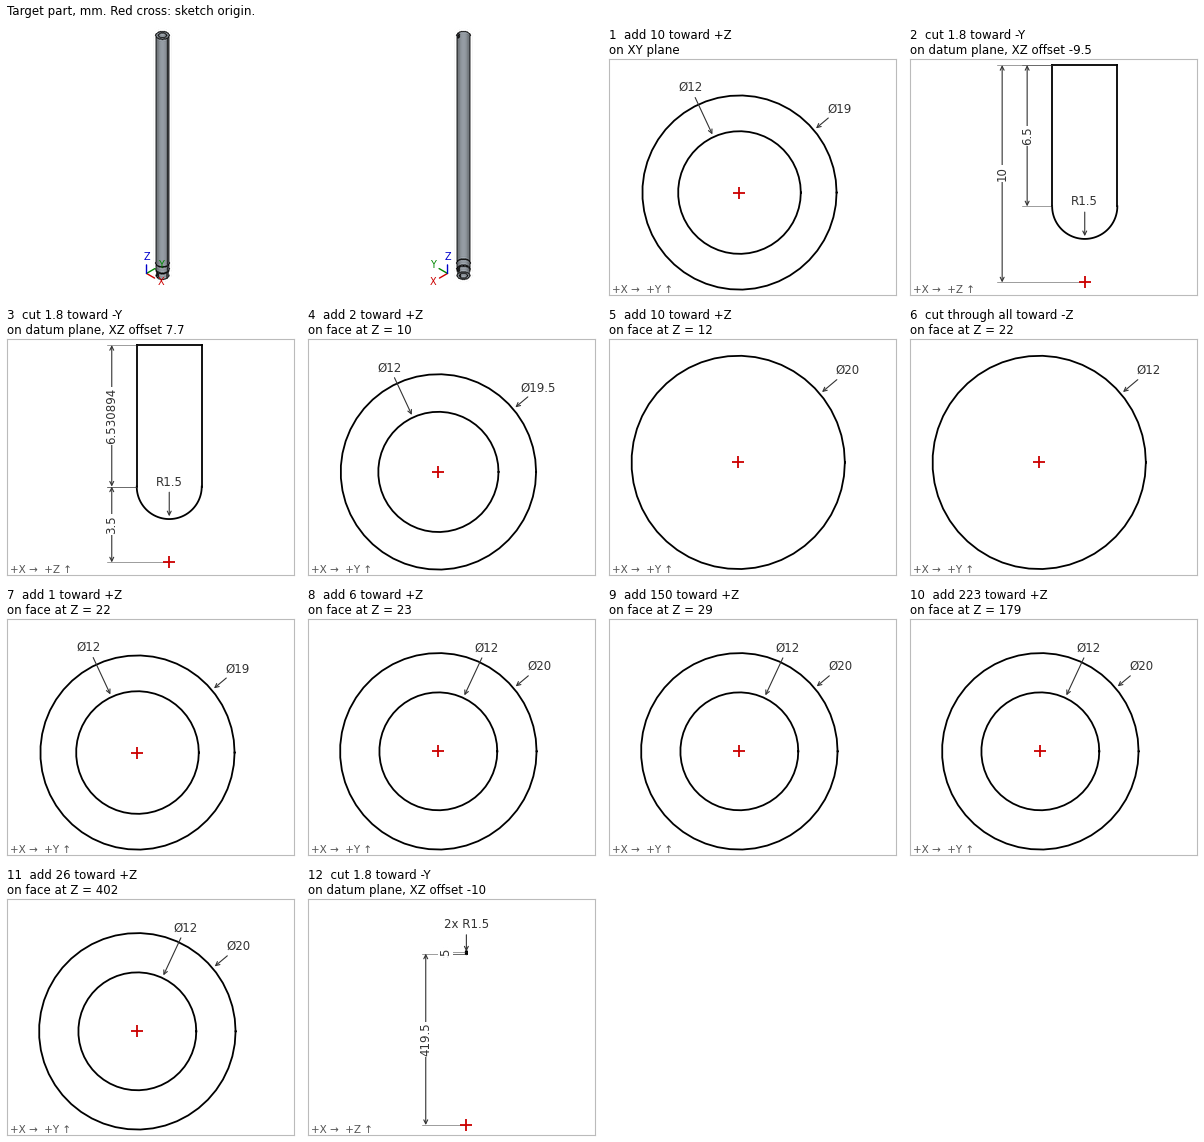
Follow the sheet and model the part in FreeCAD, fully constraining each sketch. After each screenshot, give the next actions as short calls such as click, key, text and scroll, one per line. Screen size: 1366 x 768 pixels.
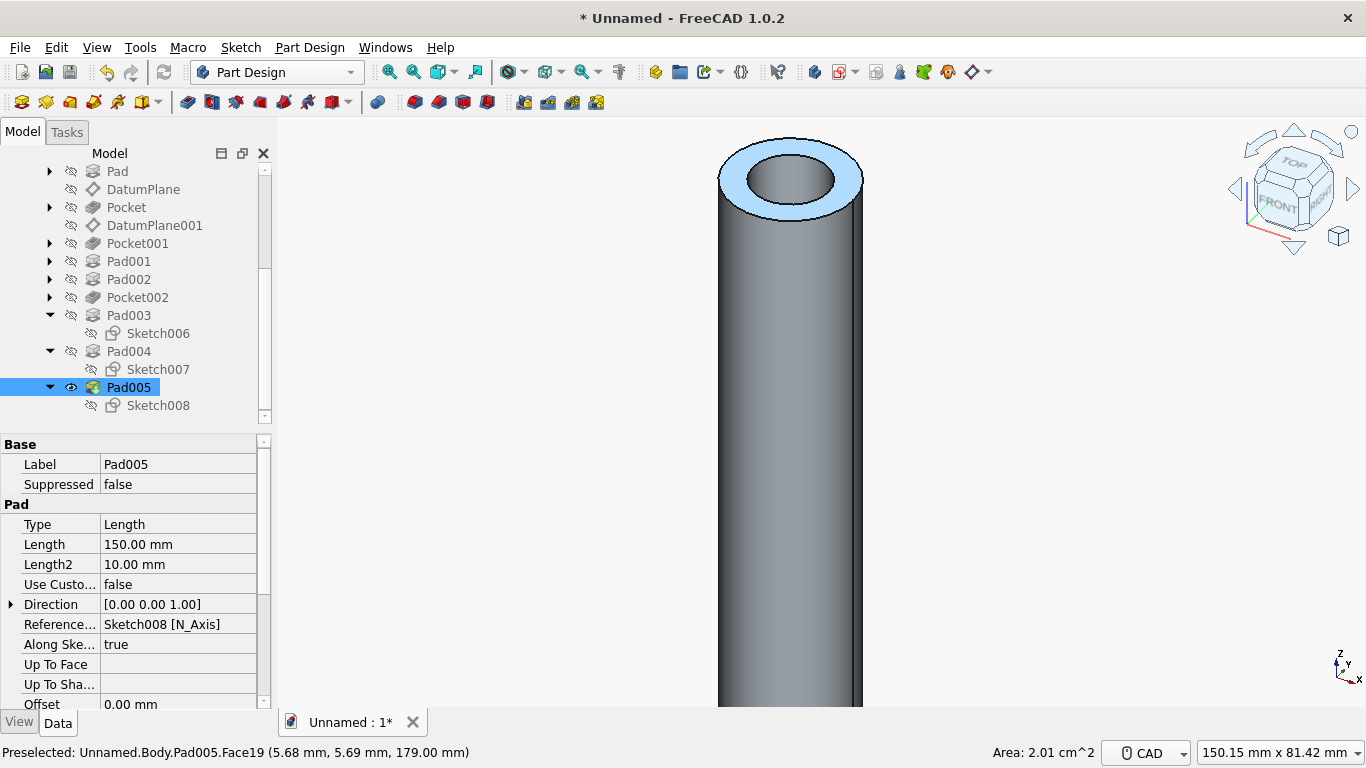
click(840, 72)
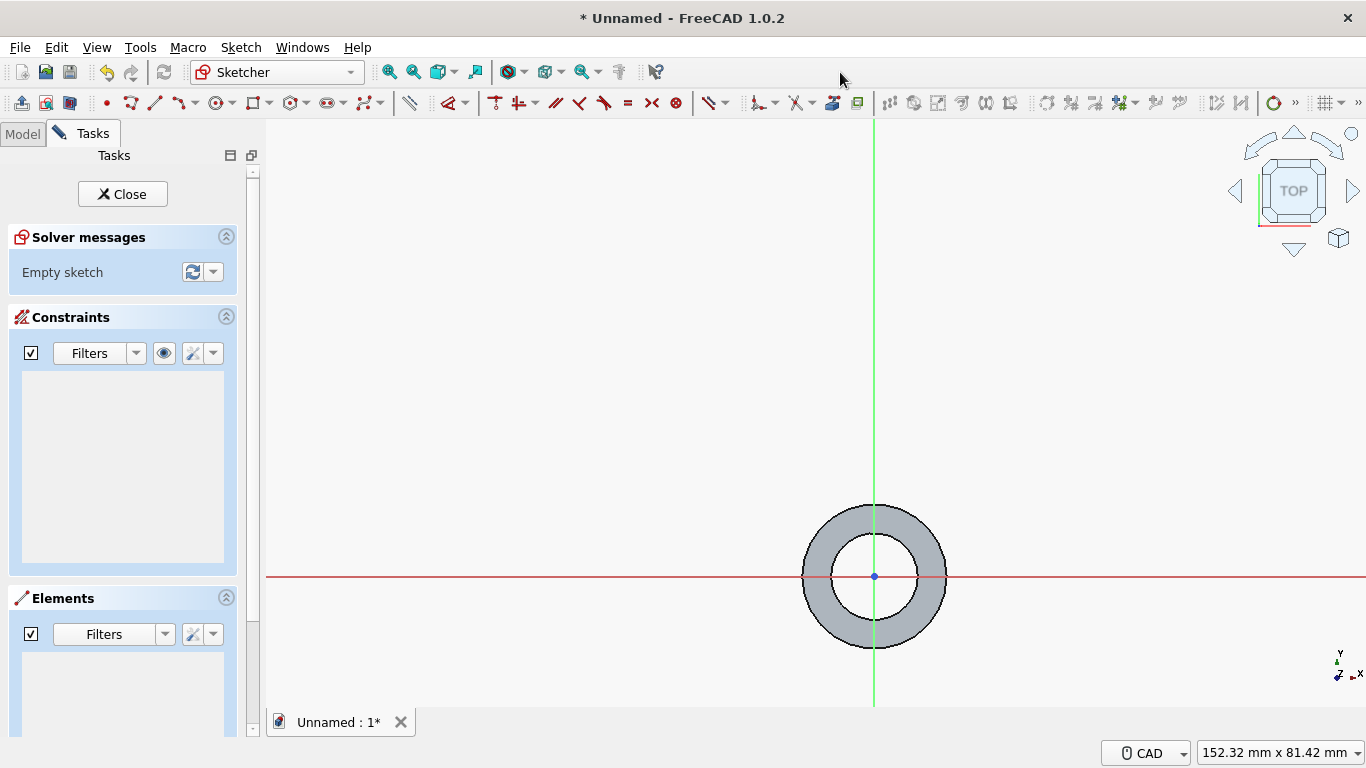
scroll(948, 672, up, 5)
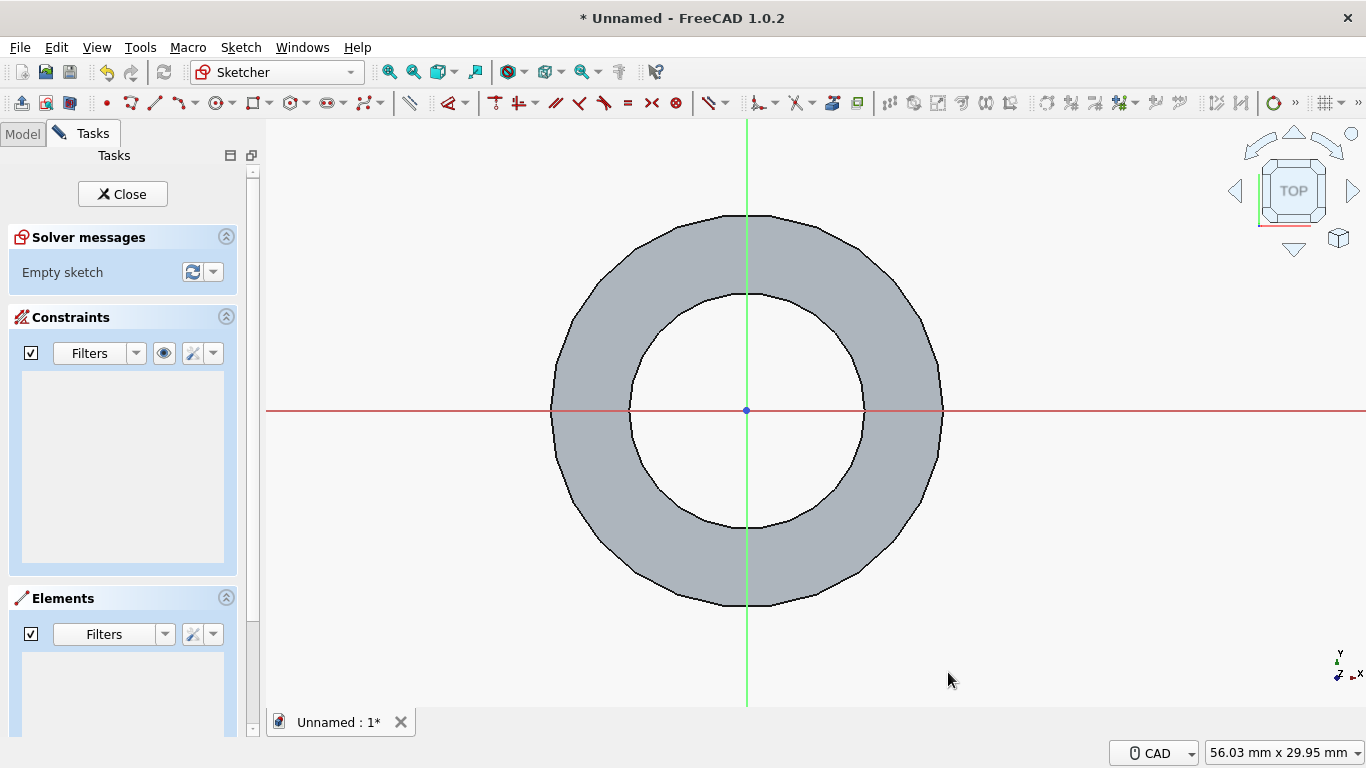
click(216, 104)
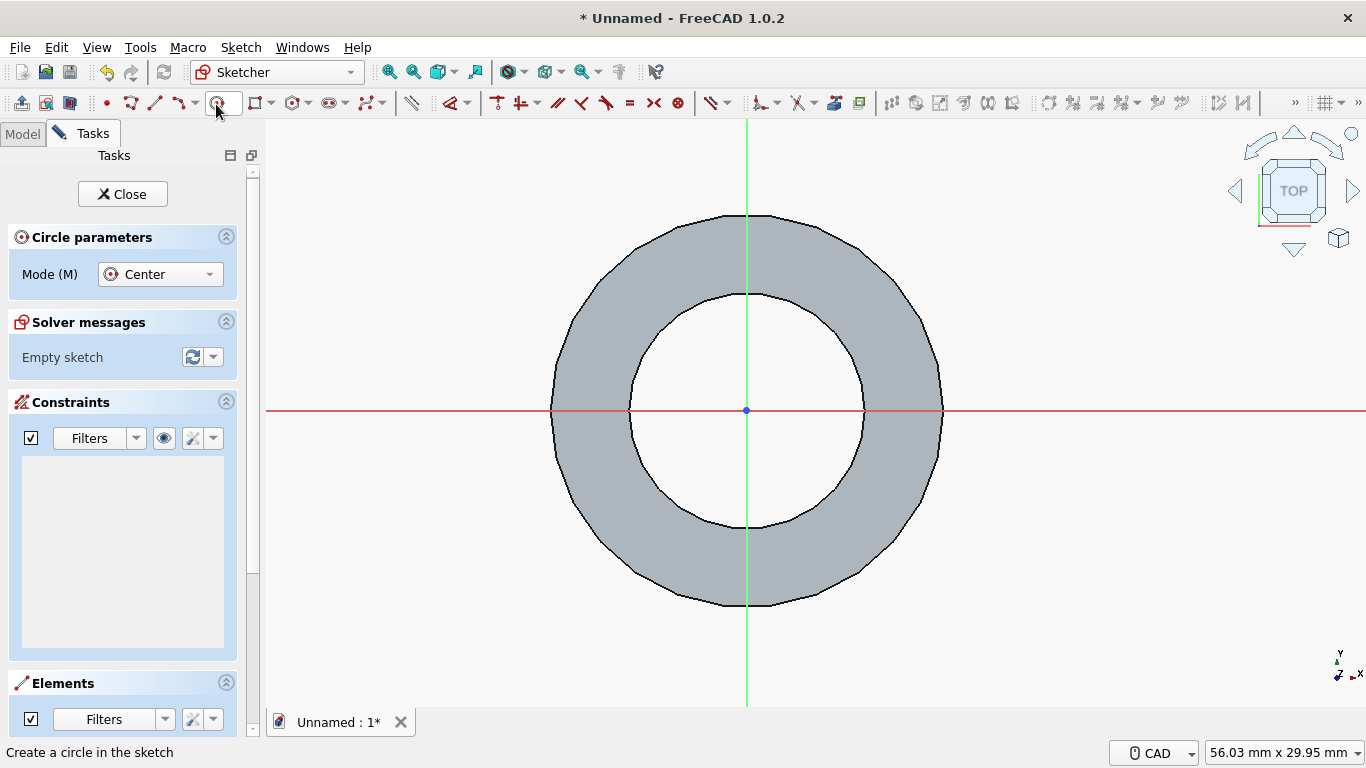
click(747, 411)
click(886, 272)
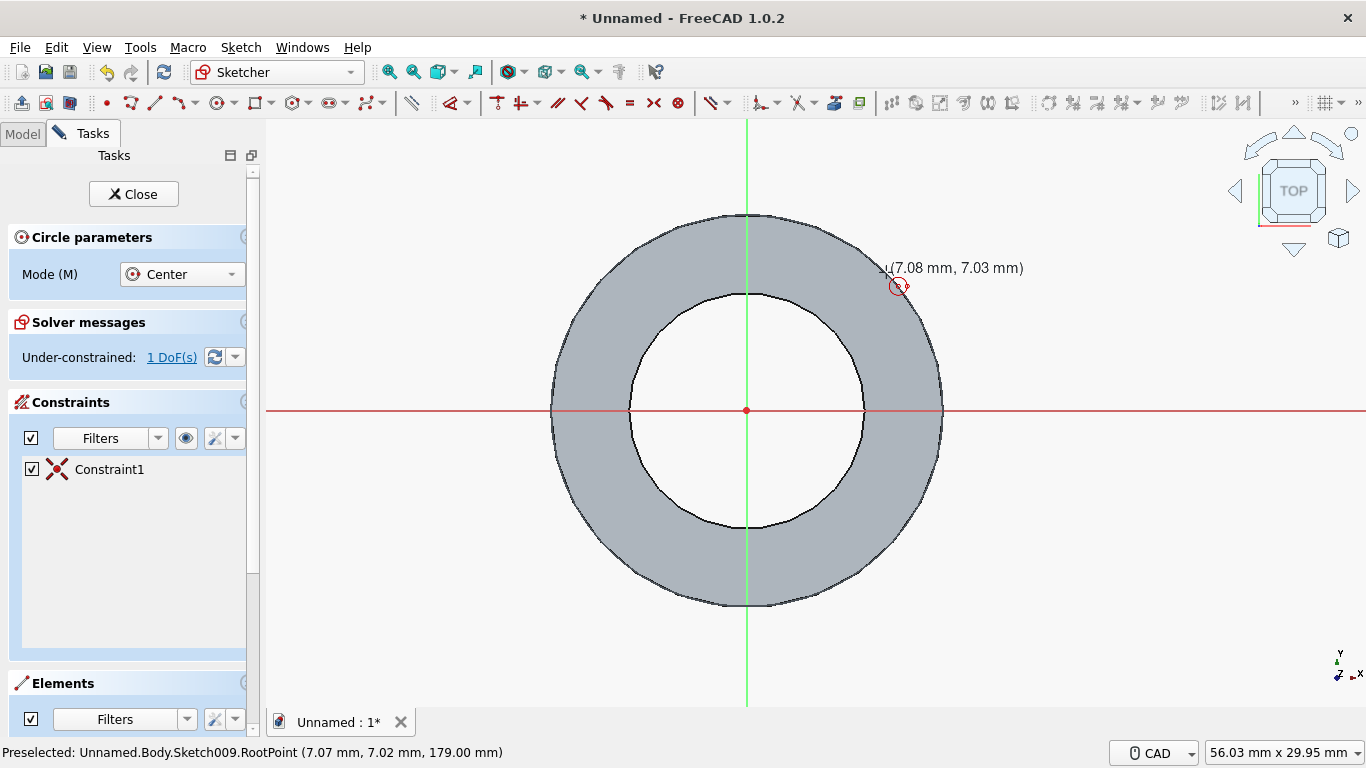
click(747, 411)
click(830, 328)
key(Escape)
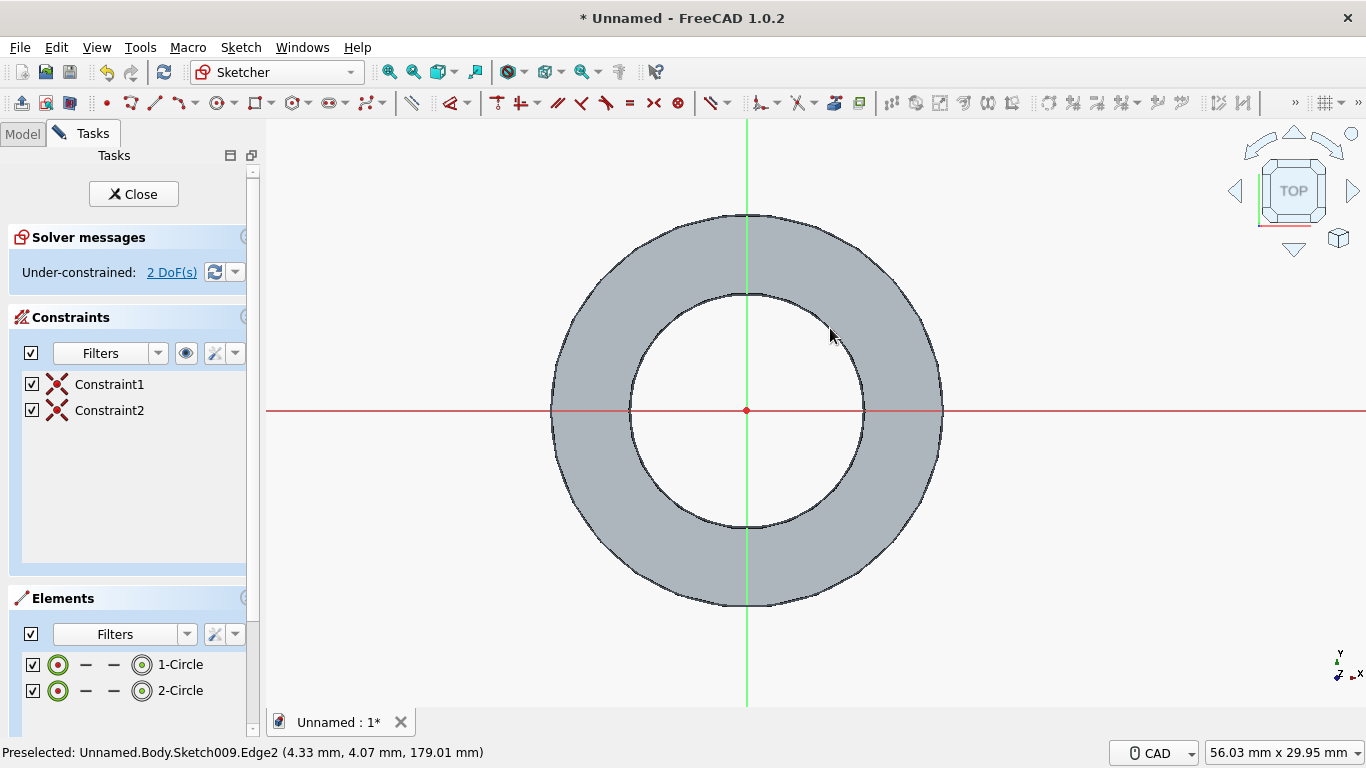
click(450, 104)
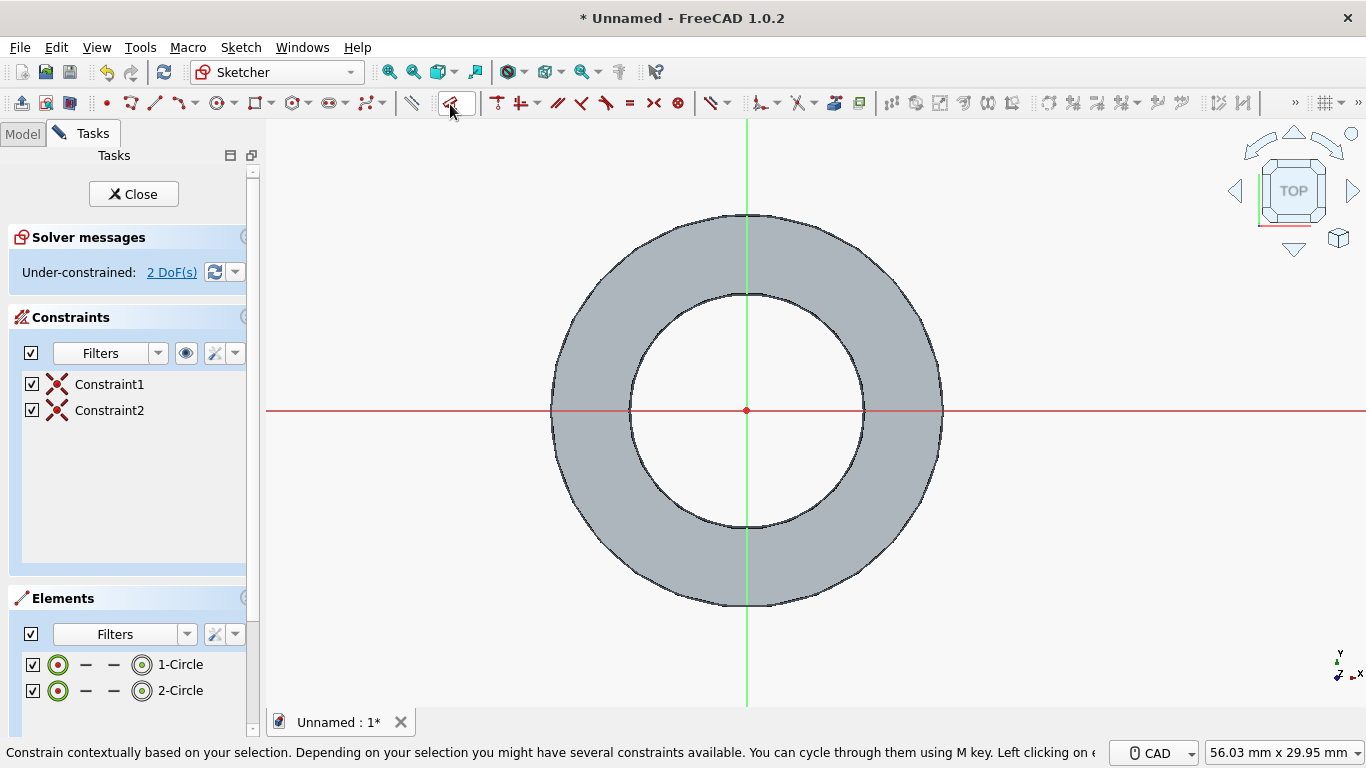
click(885, 272)
click(908, 249)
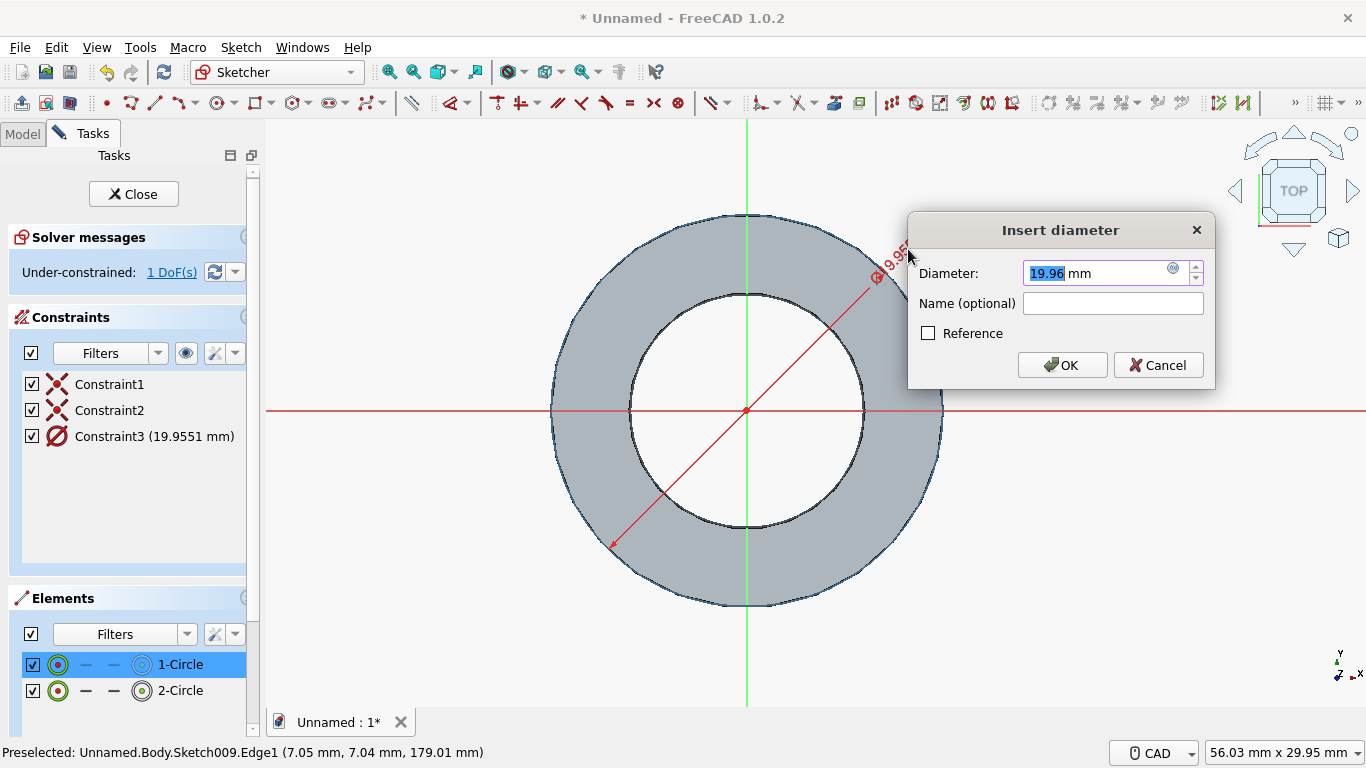
text(20)
key(Return)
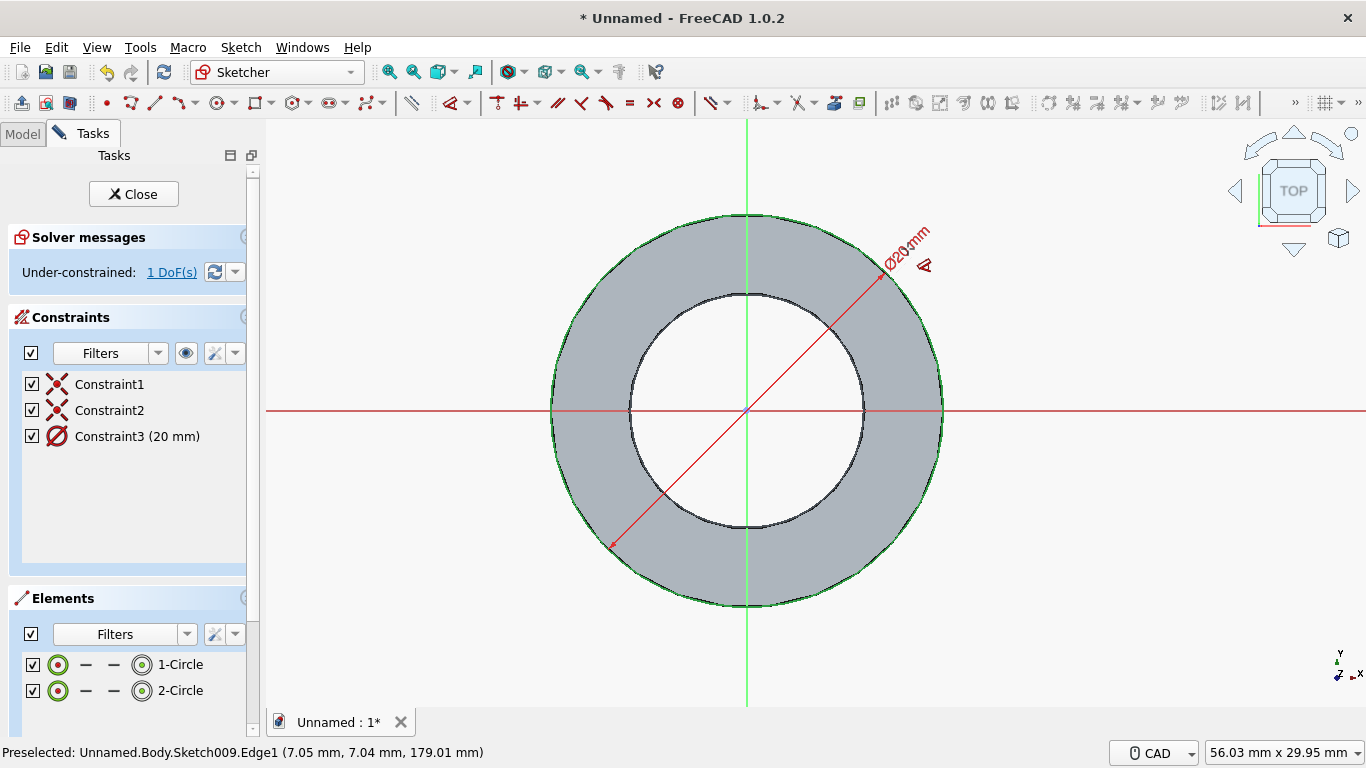
click(829, 328)
click(851, 305)